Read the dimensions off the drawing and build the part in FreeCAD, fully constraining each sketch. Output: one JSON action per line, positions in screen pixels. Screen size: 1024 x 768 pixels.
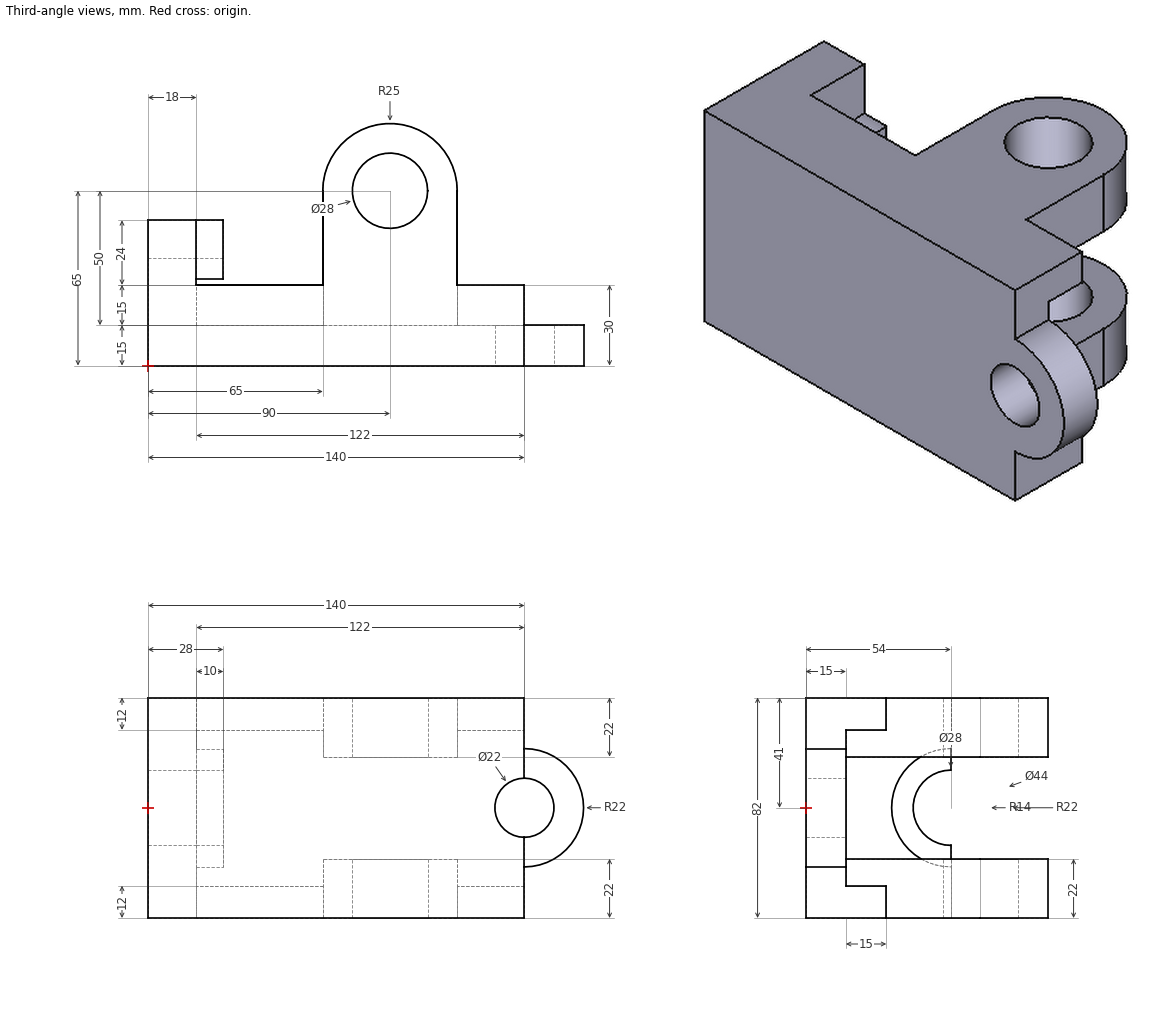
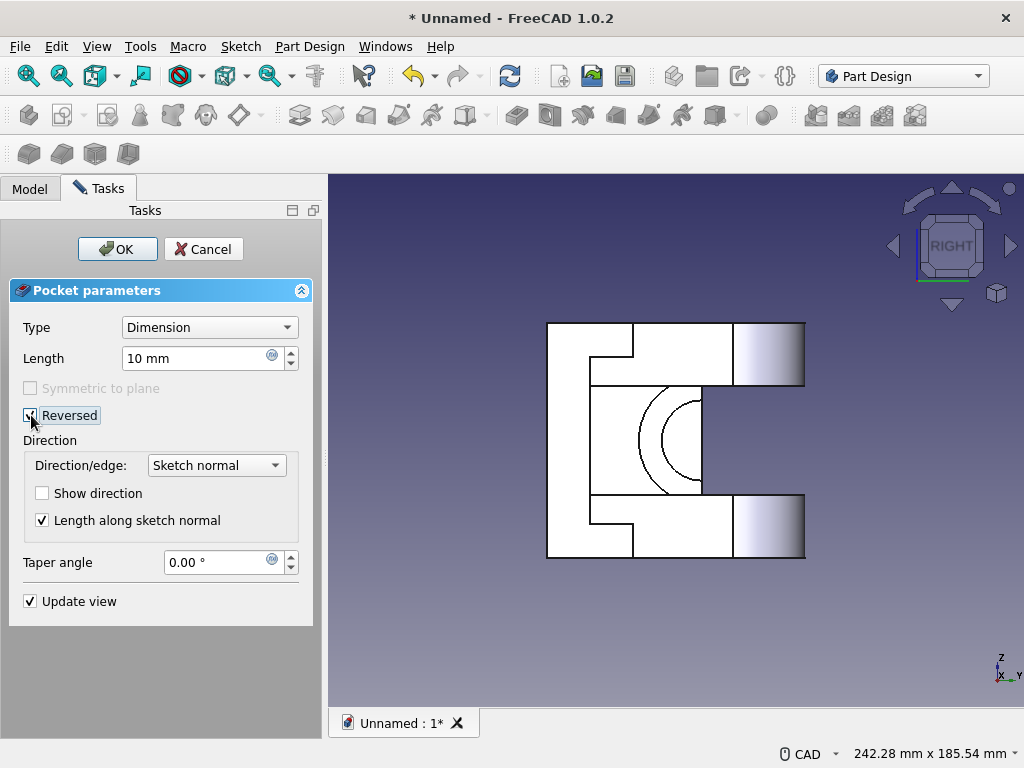
{"action": "left_click", "coordinate": [118, 249]}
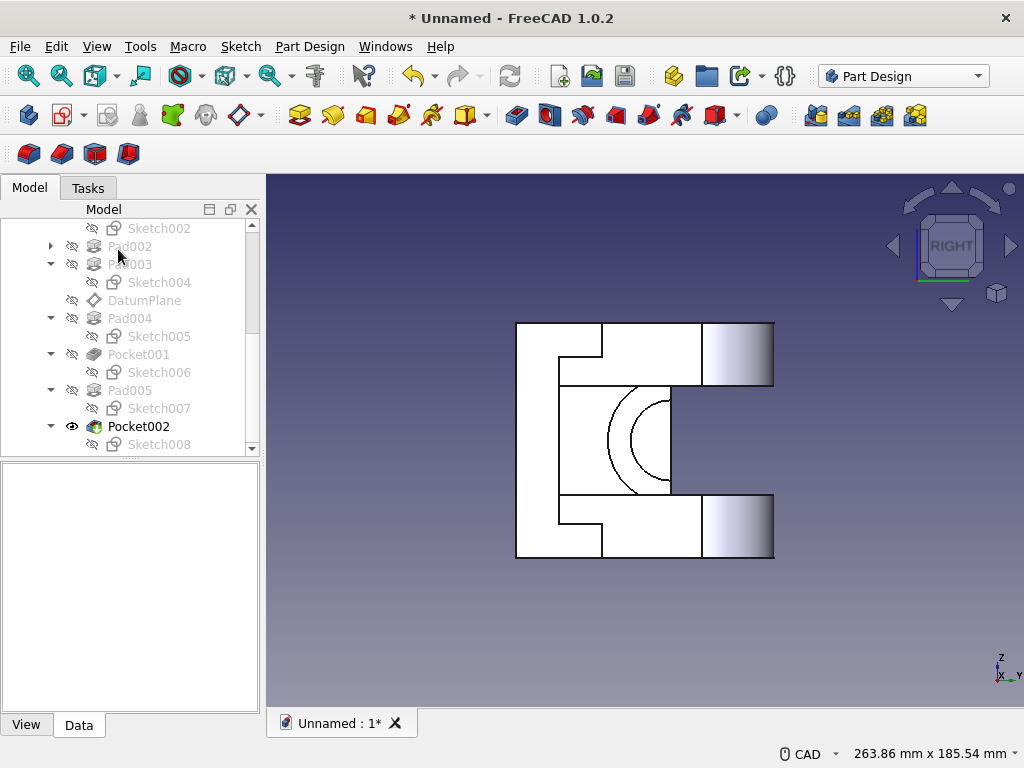
{"action": "key", "text": "v f"}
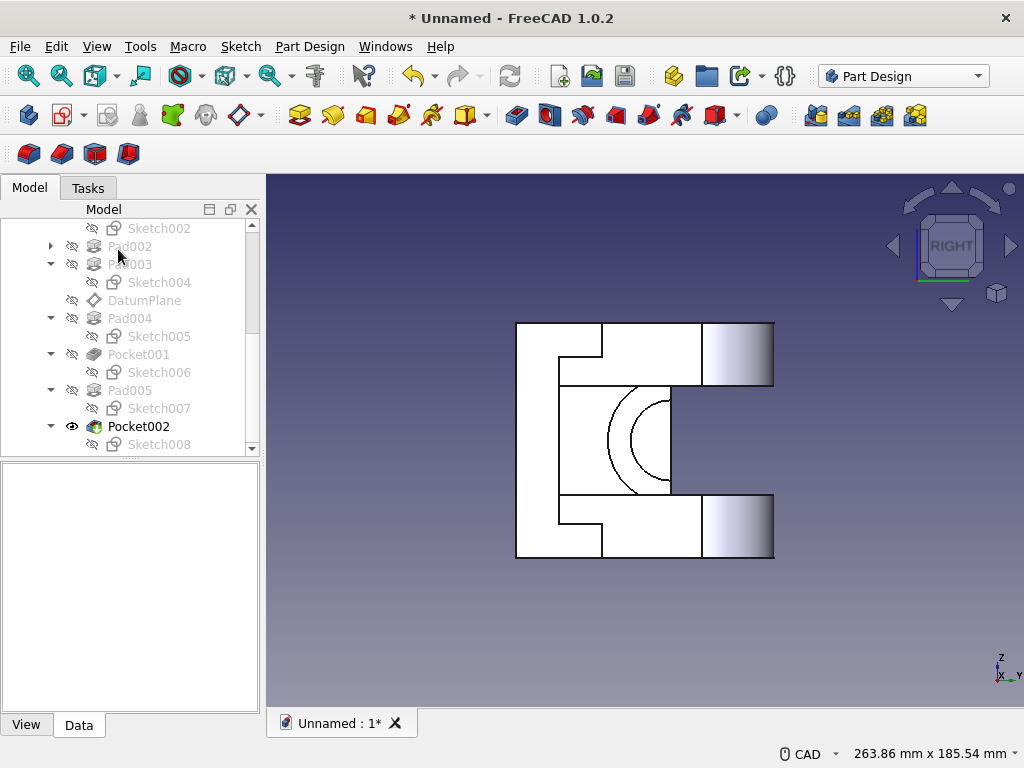
{"action": "key", "text": "6"}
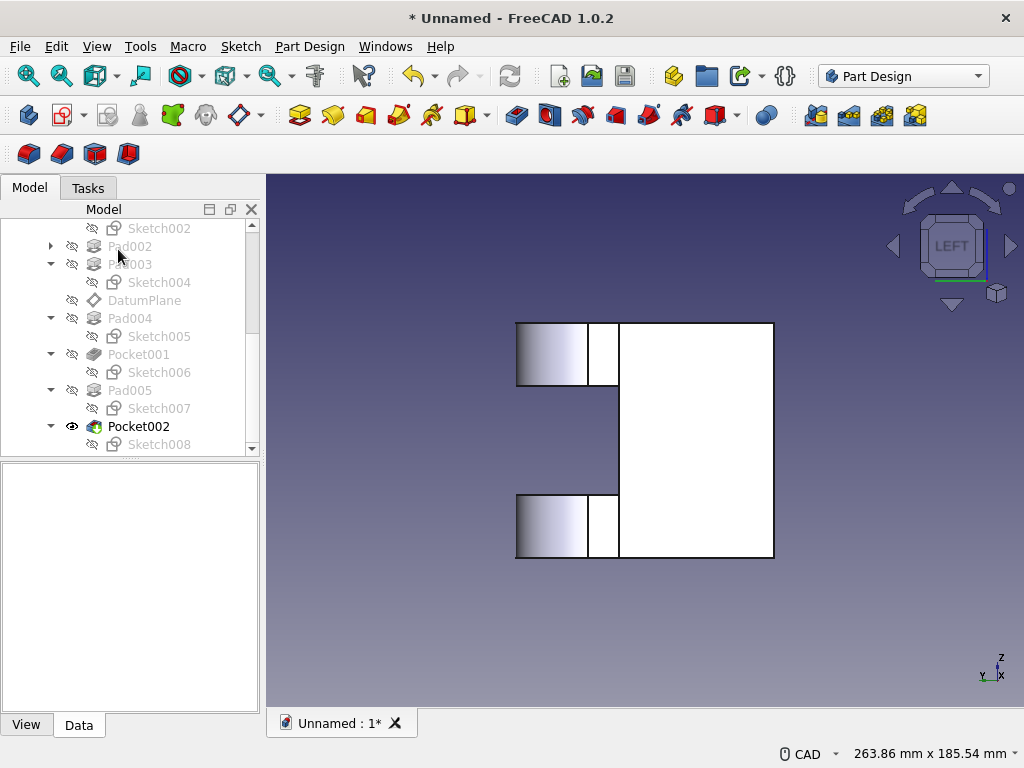
{"action": "key", "text": "v f"}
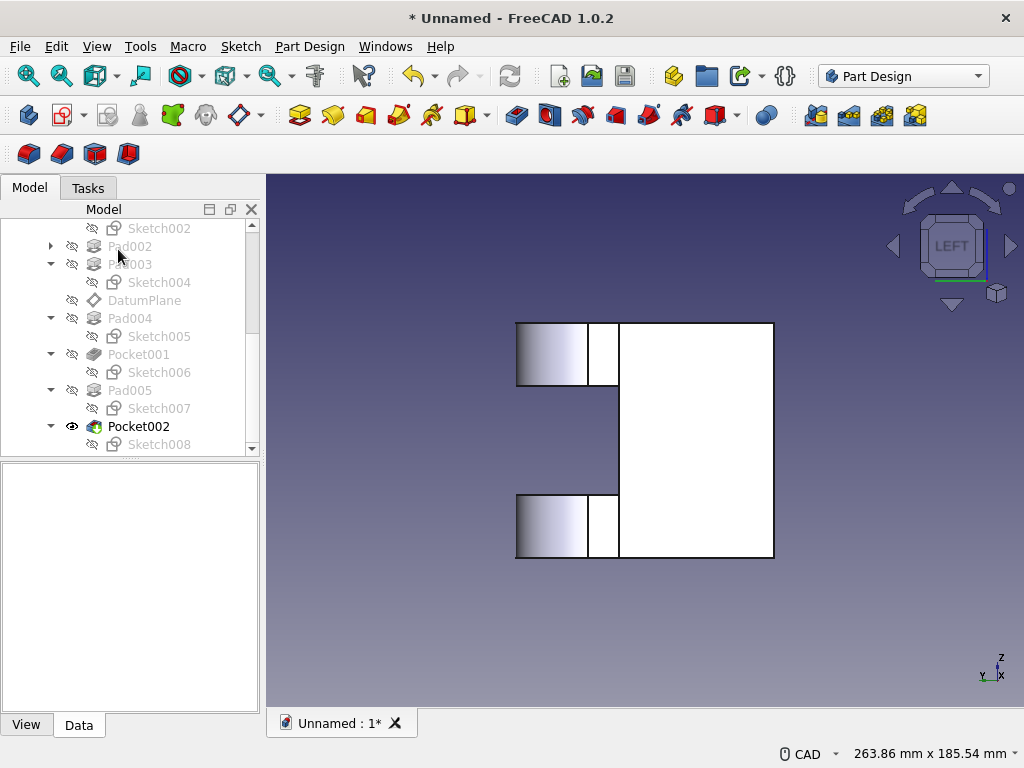
{"action": "left_click", "coordinate": [697, 406]}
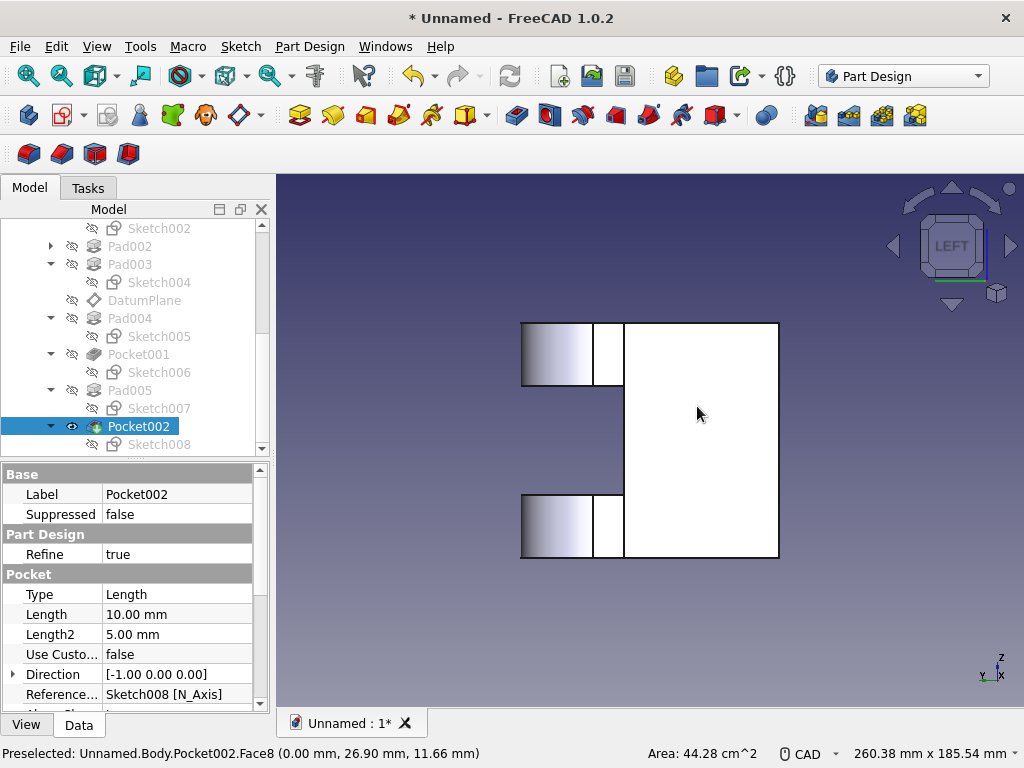
{"action": "left_click", "coordinate": [62, 116]}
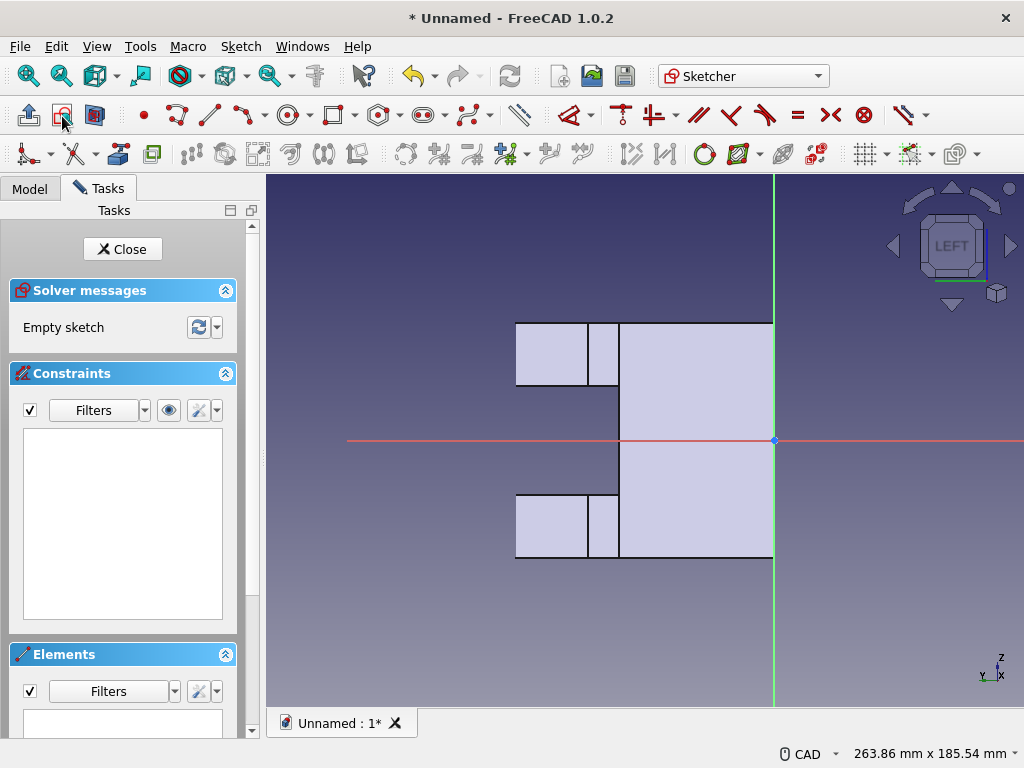
{"action": "scroll", "coordinate": [758, 440], "scroll_direction": "up", "scroll_amount": 4}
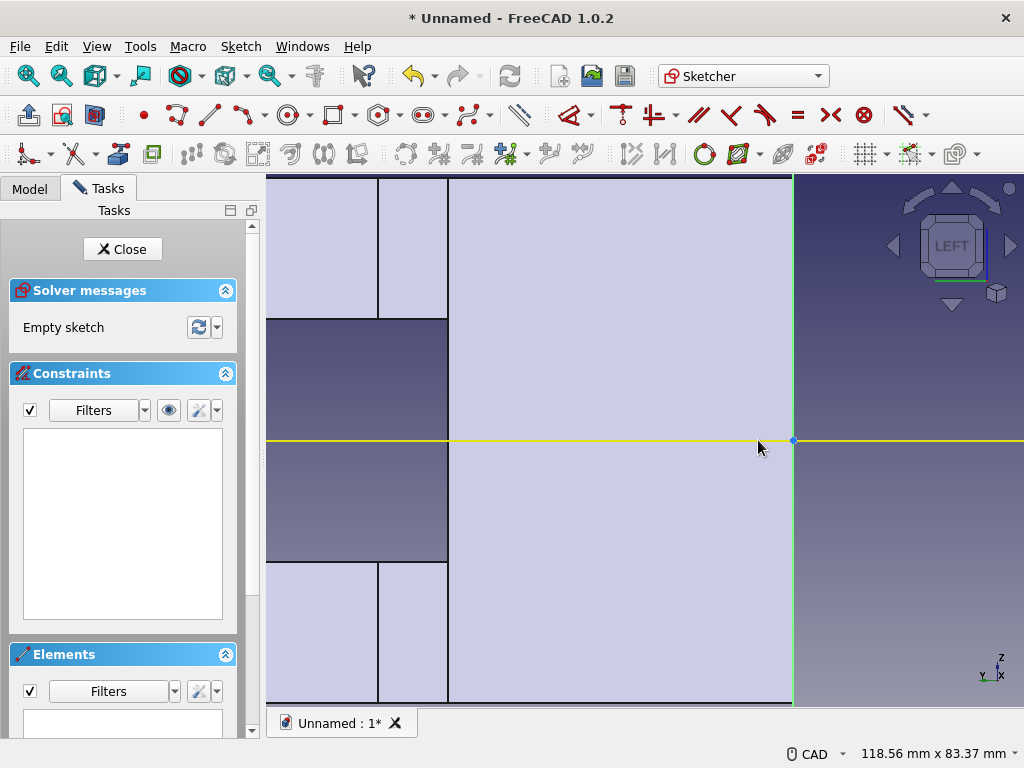
{"action": "key", "text": "g c"}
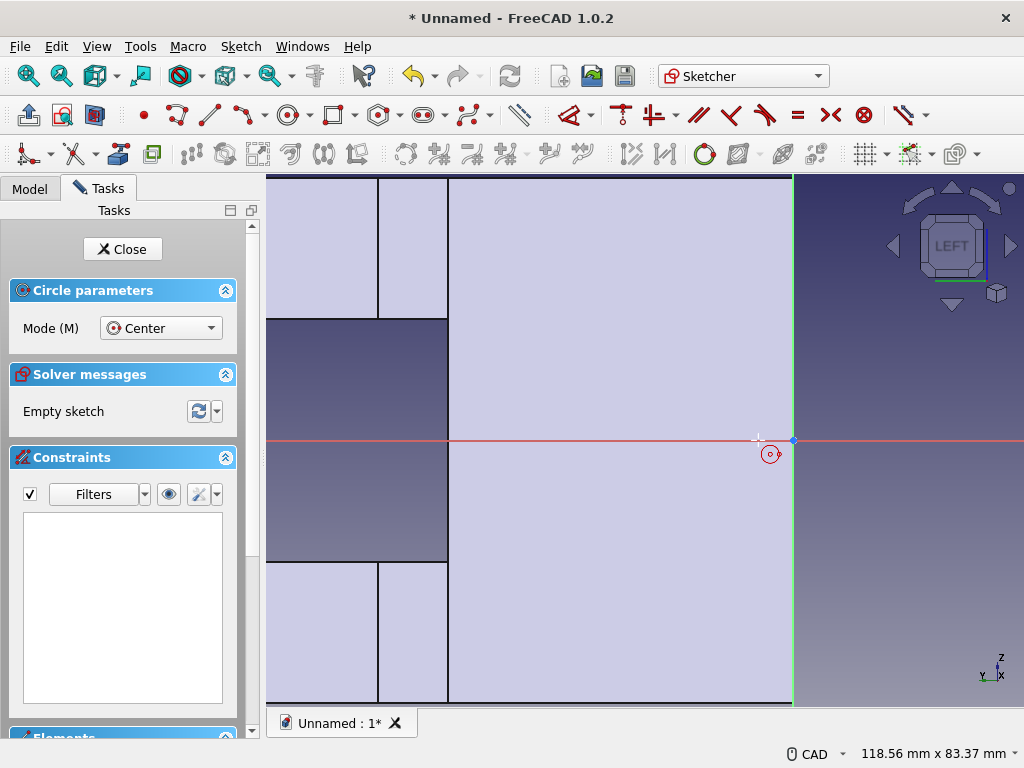
{"action": "left_click", "coordinate": [448, 440]}
{"action": "left_click", "coordinate": [511, 377]}
{"action": "key", "text": "Escape"}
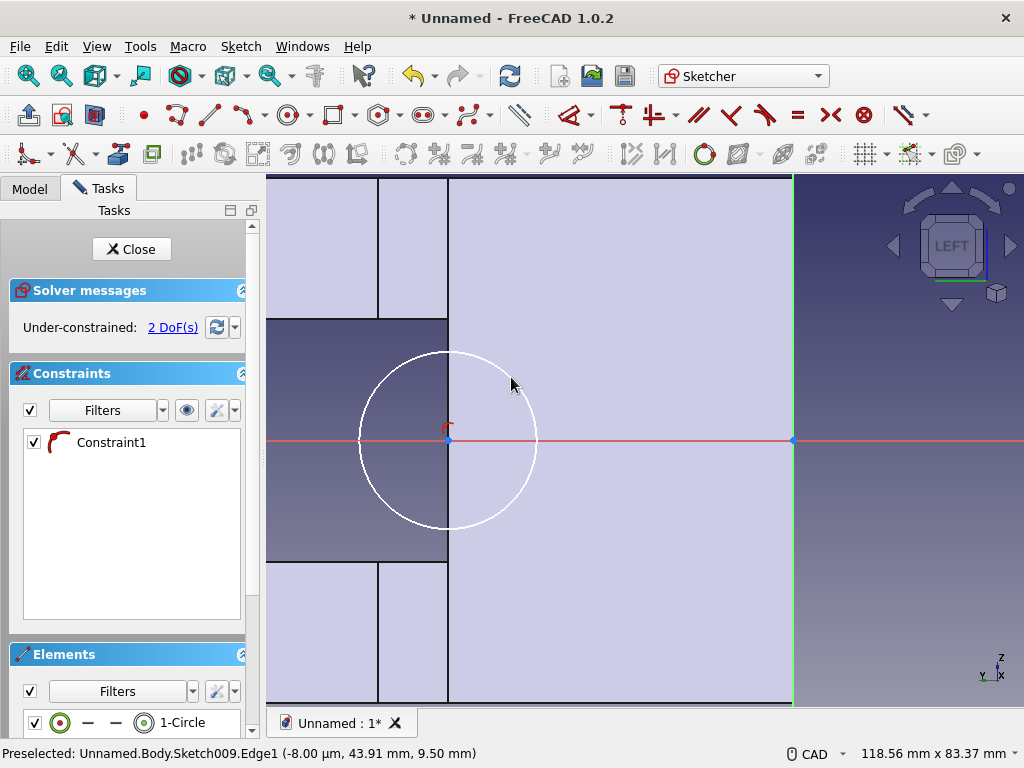
{"action": "left_click", "coordinate": [568, 116]}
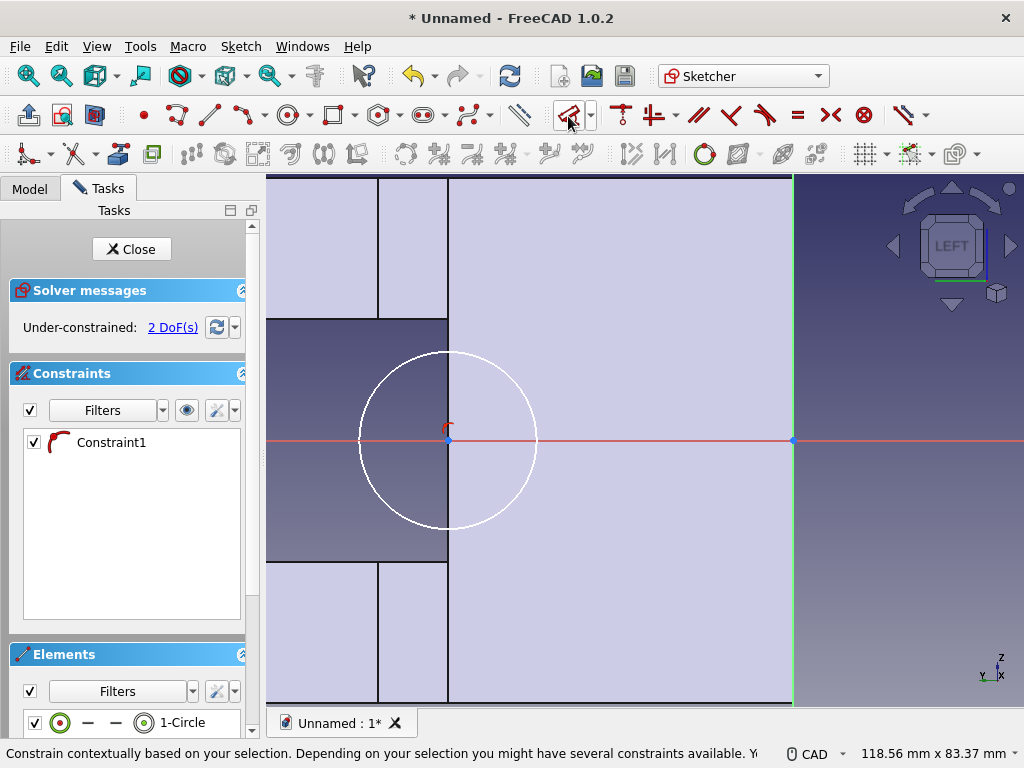
{"action": "left_click", "coordinate": [511, 378]}
{"action": "left_click", "coordinate": [534, 355]}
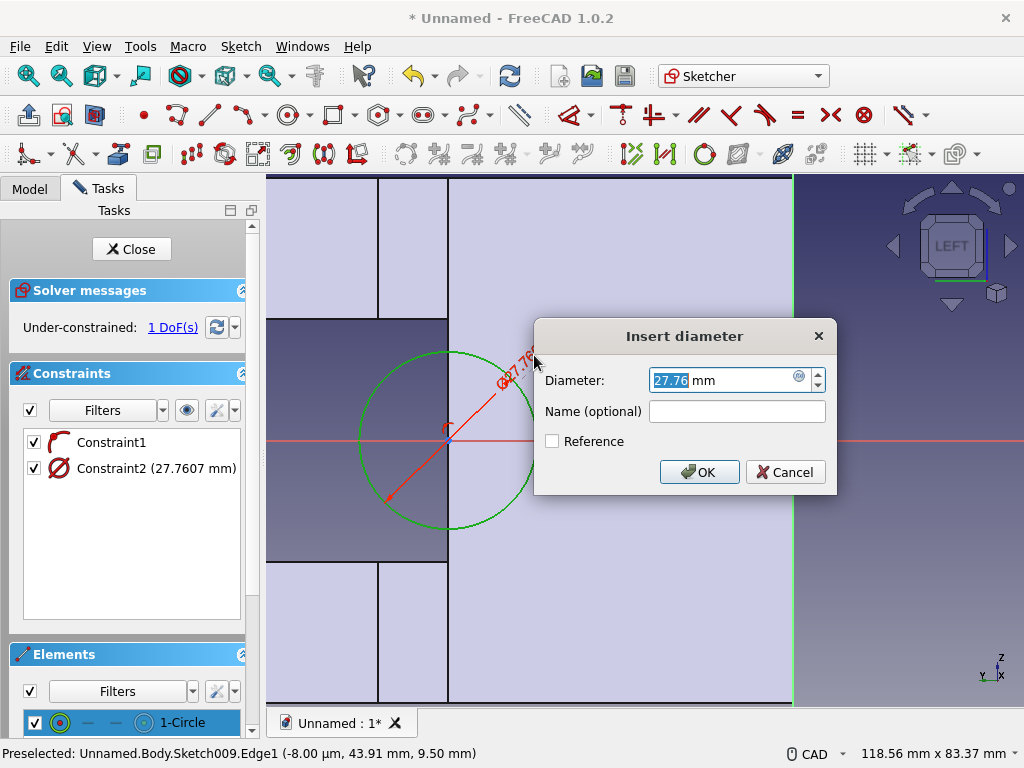
{"action": "type", "text": "28"}
{"action": "key", "text": "Return"}